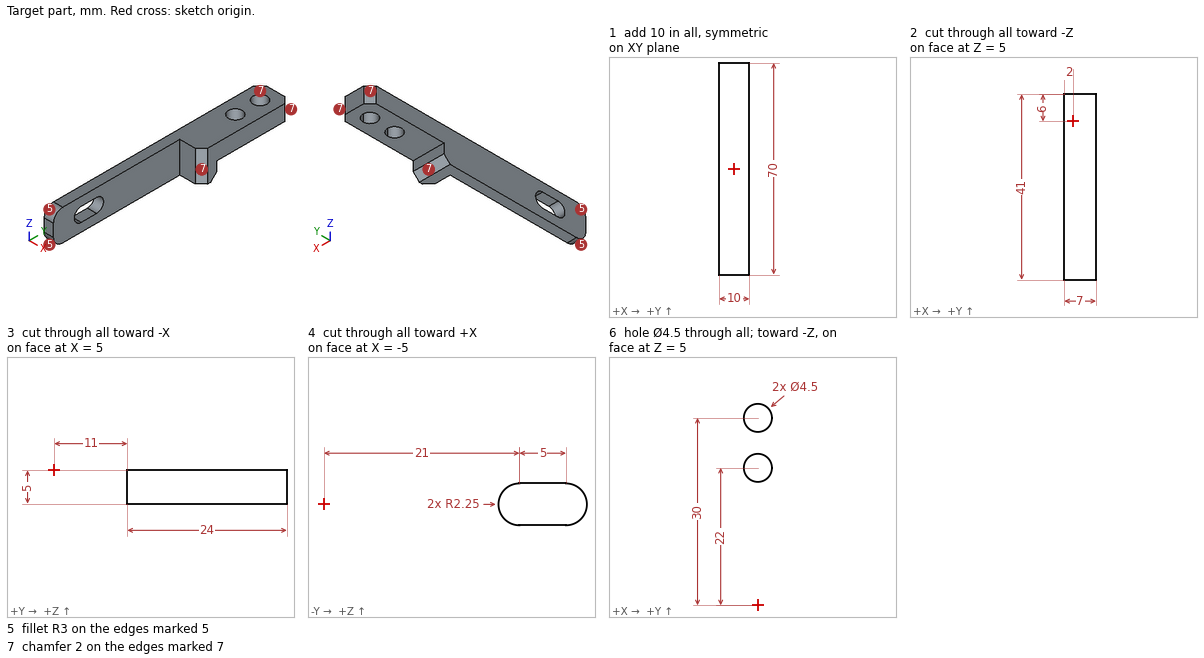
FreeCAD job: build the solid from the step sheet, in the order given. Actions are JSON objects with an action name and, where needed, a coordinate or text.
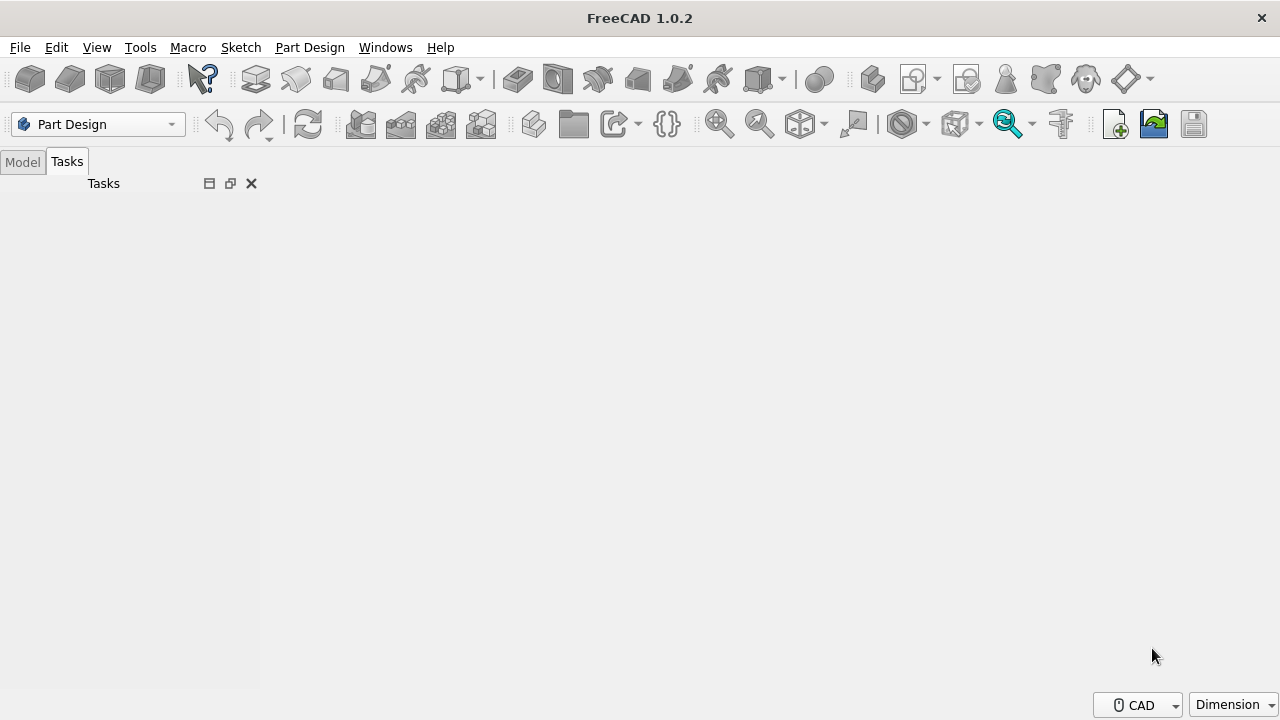
{"action": "key", "text": "ctrl+n"}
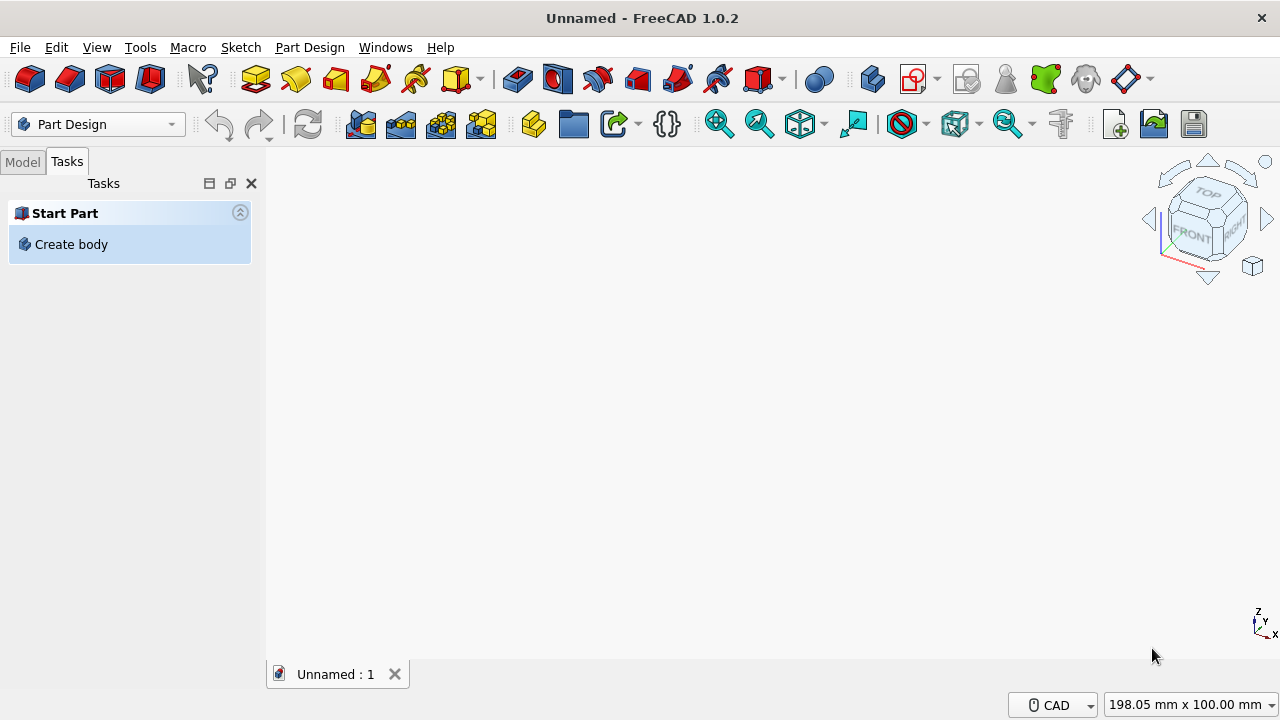
{"action": "left_click", "coordinate": [914, 80]}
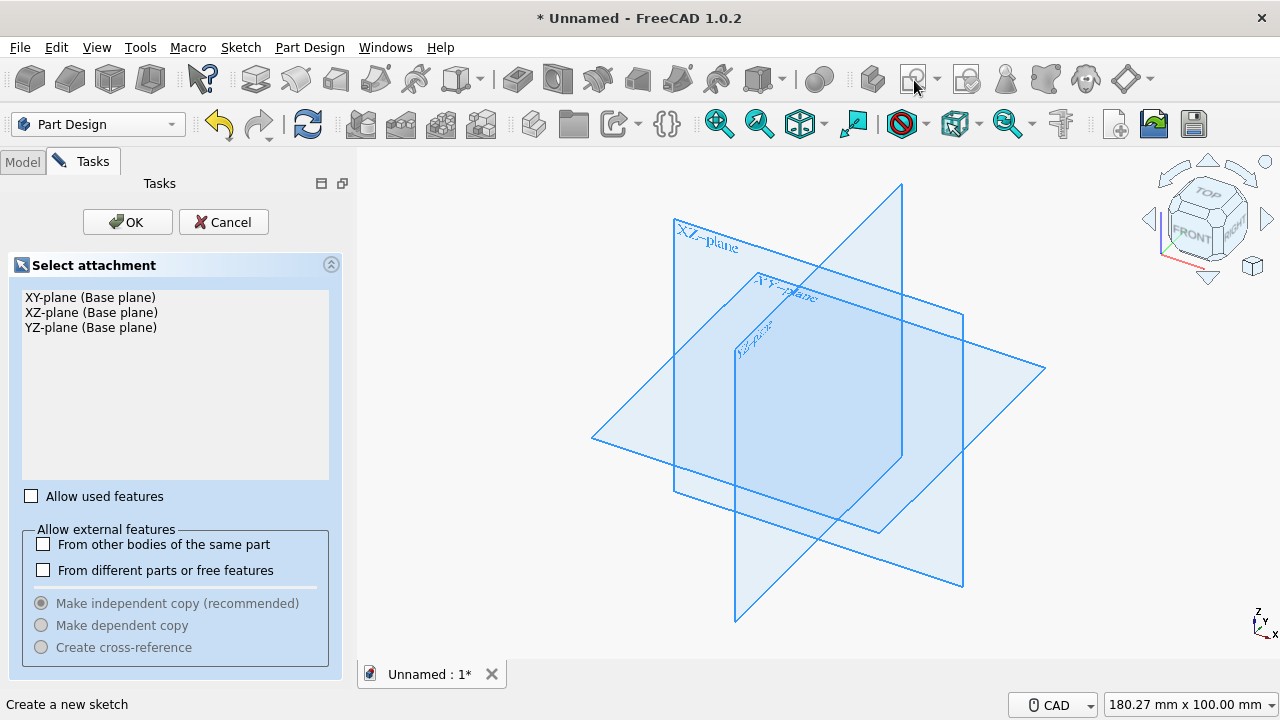
{"action": "left_click", "coordinate": [82, 298]}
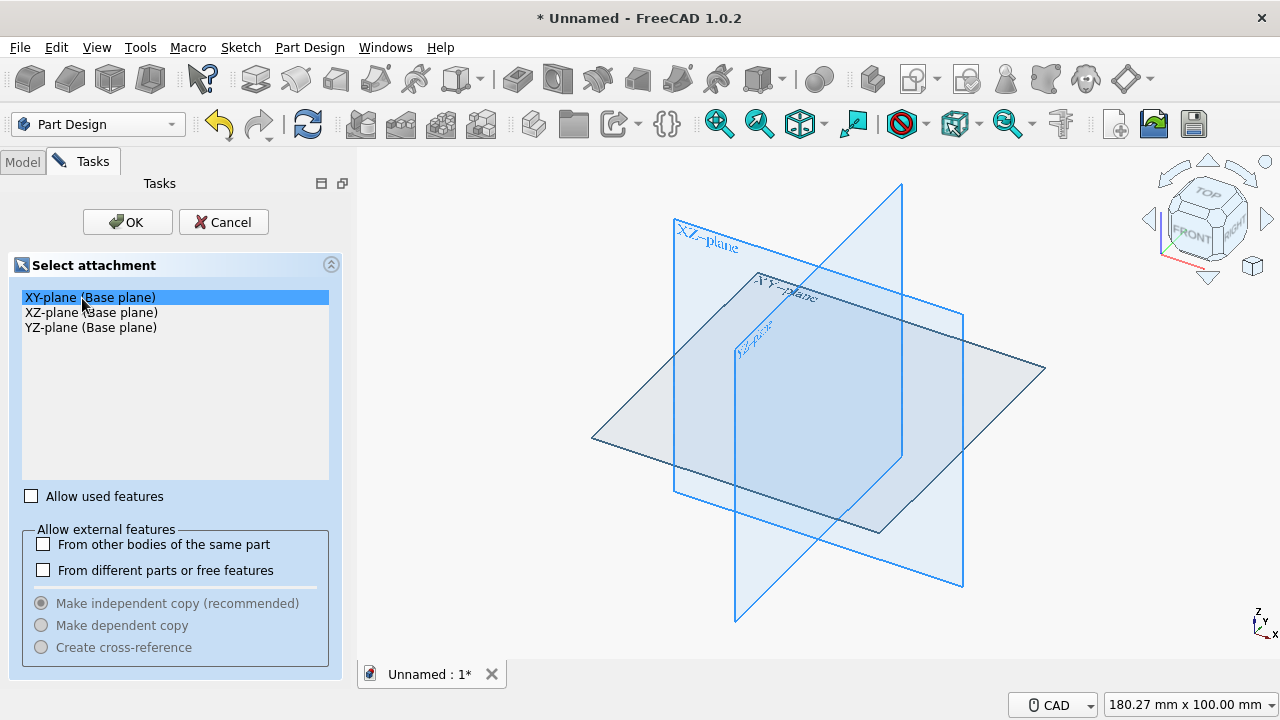
{"action": "left_click", "coordinate": [128, 222]}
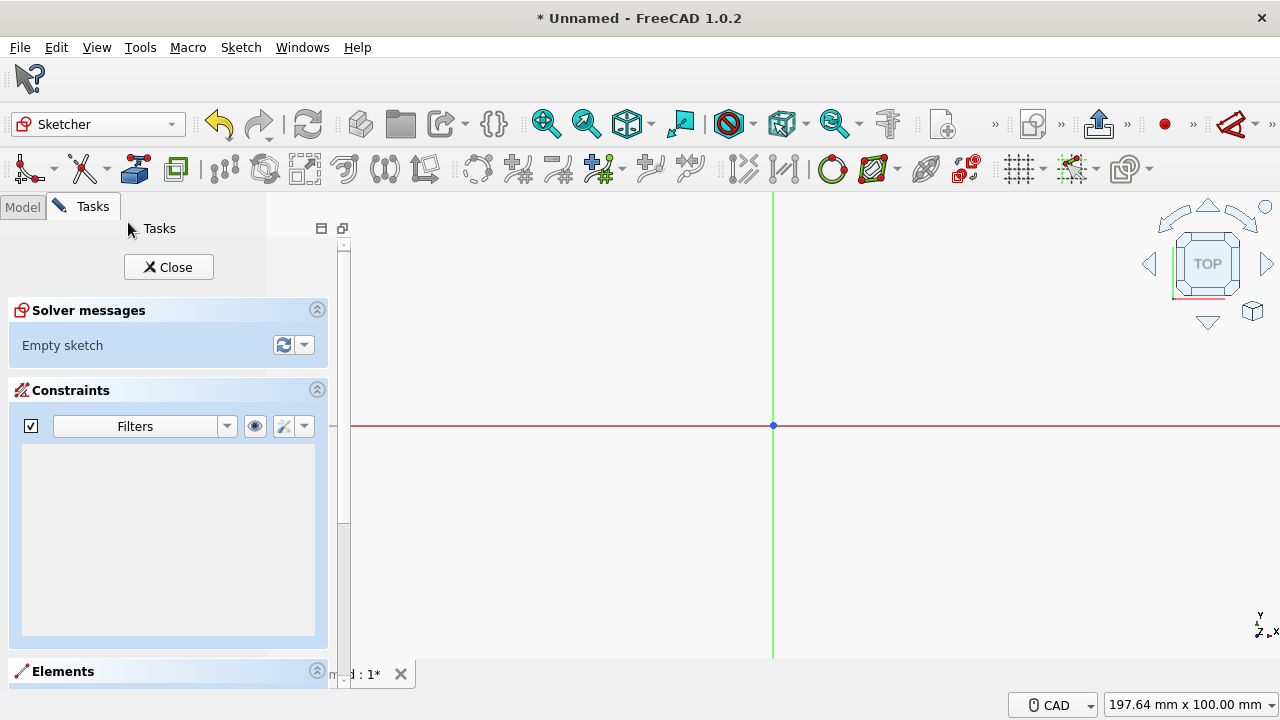
{"action": "key", "text": "g v"}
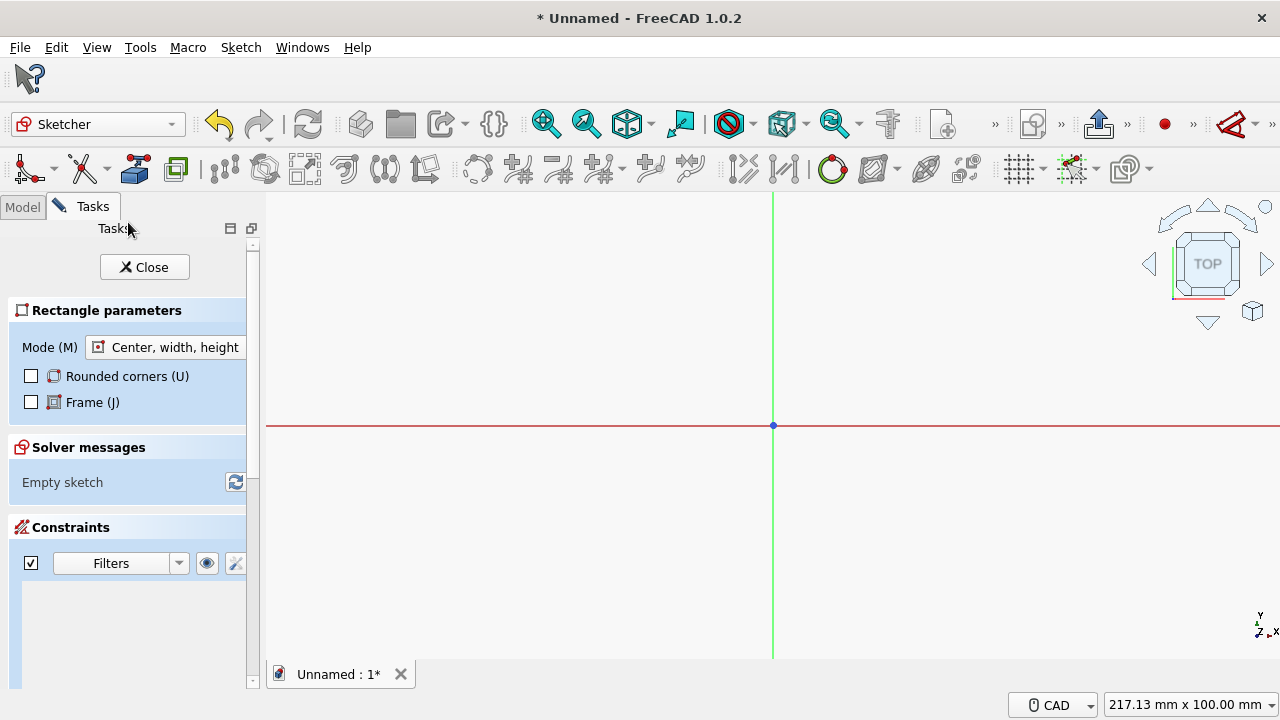
{"action": "left_click", "coordinate": [773, 426]}
{"action": "left_click", "coordinate": [796, 262]}
{"action": "key", "text": "Escape"}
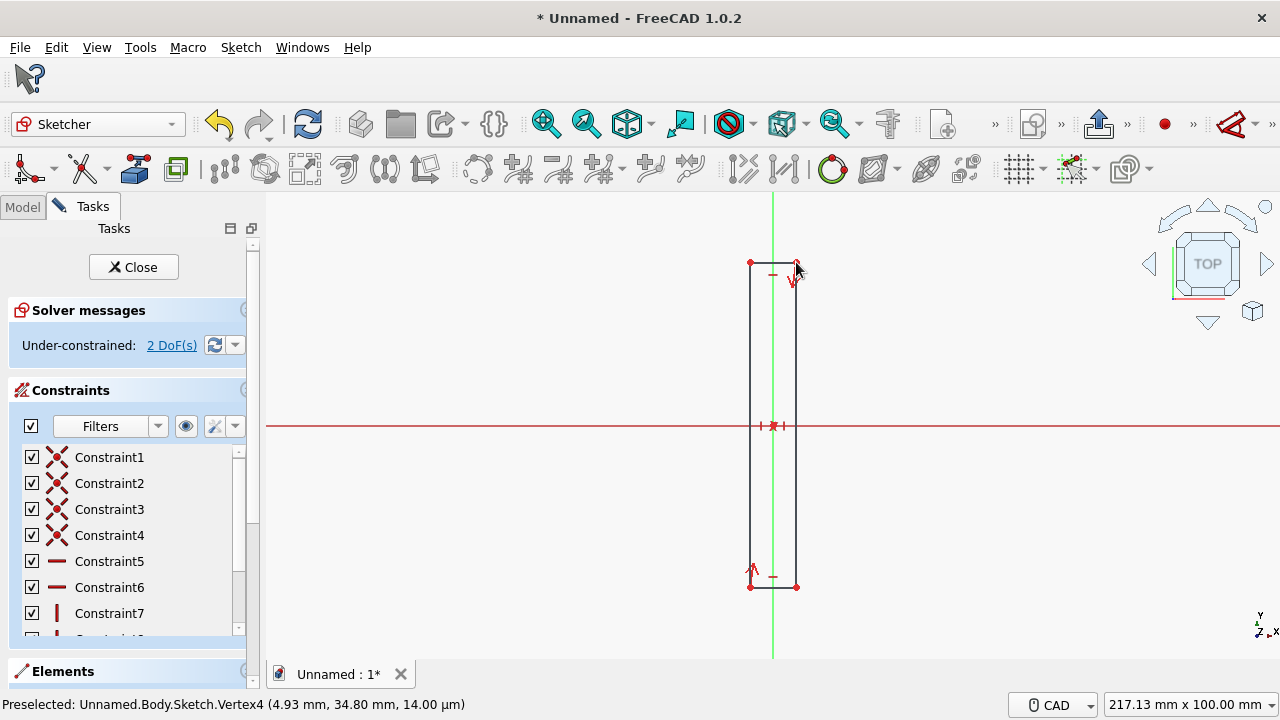
{"action": "key", "text": "d"}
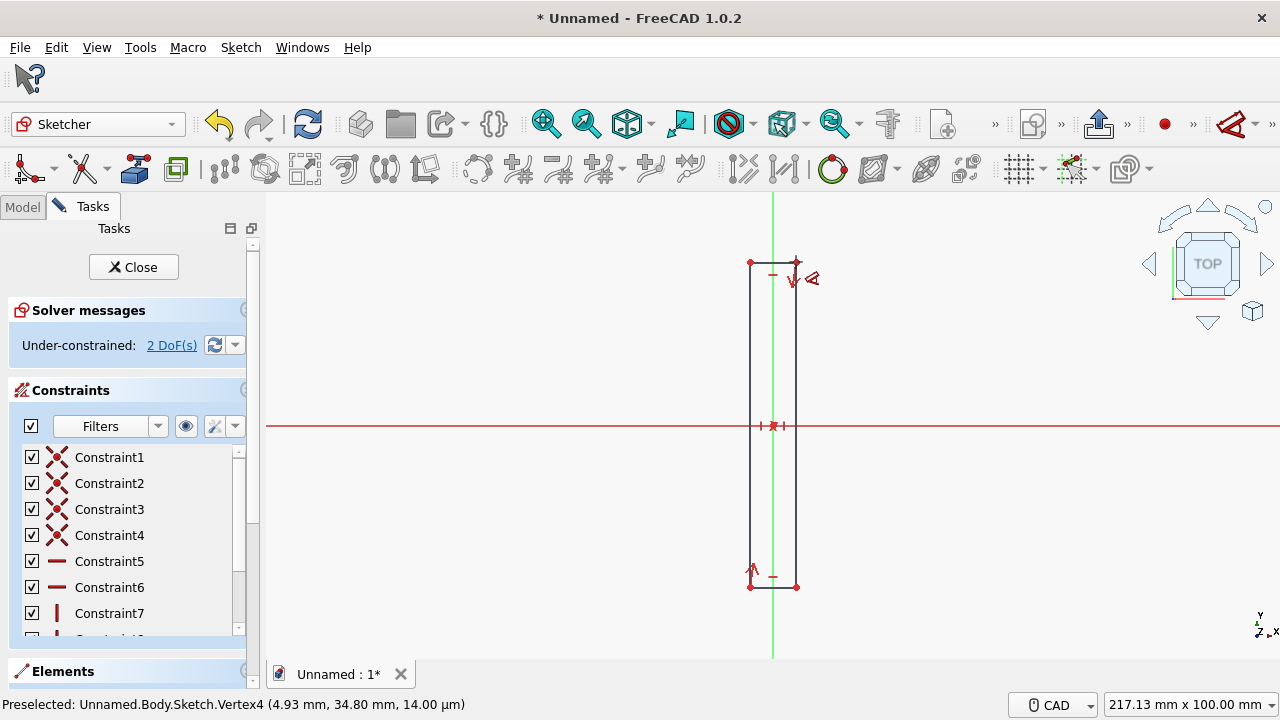
{"action": "scroll", "coordinate": [764, 588], "scroll_direction": "up", "scroll_amount": 3}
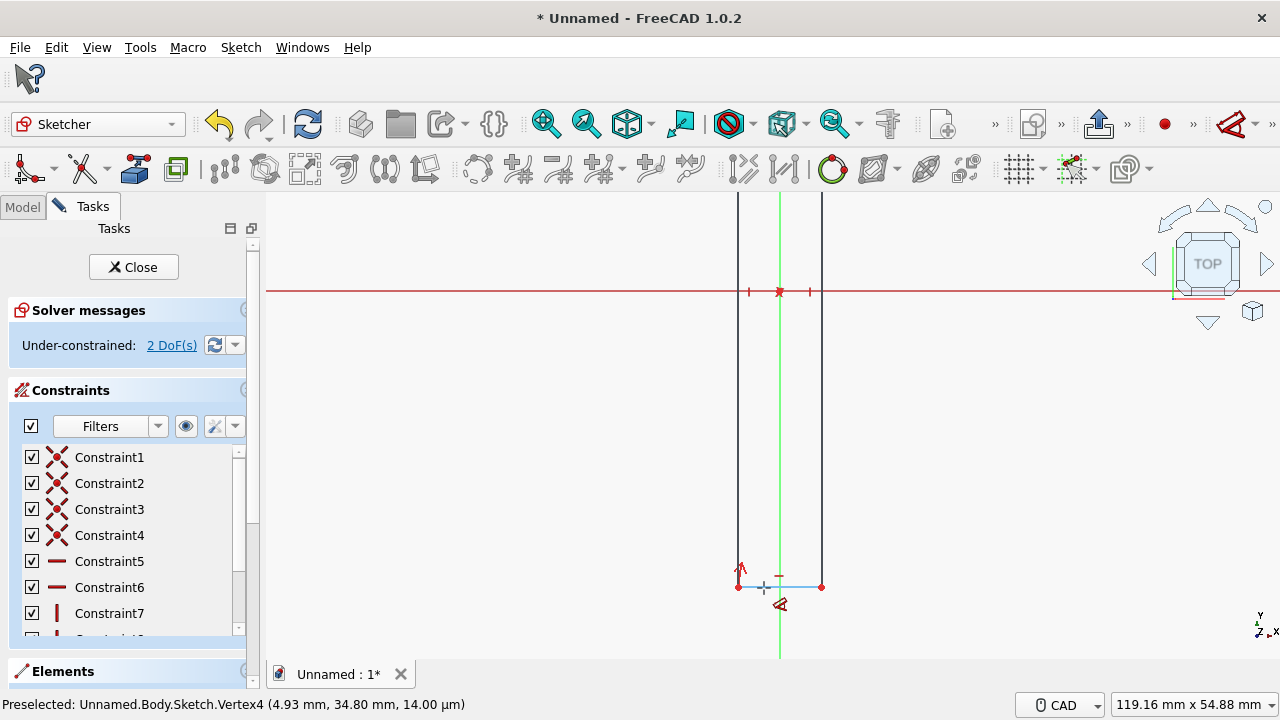
{"action": "left_click", "coordinate": [763, 587]}
{"action": "left_click", "coordinate": [761, 621]}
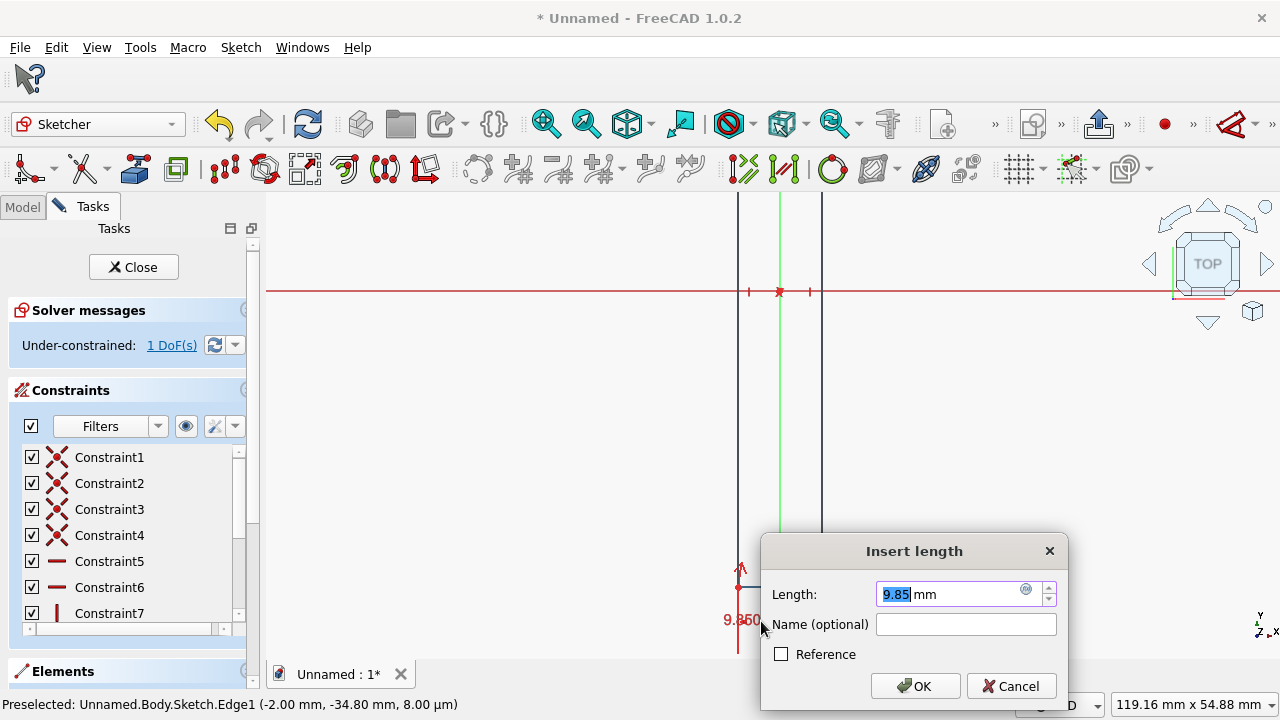
{"action": "type", "text": "10"}
{"action": "key", "text": "Return"}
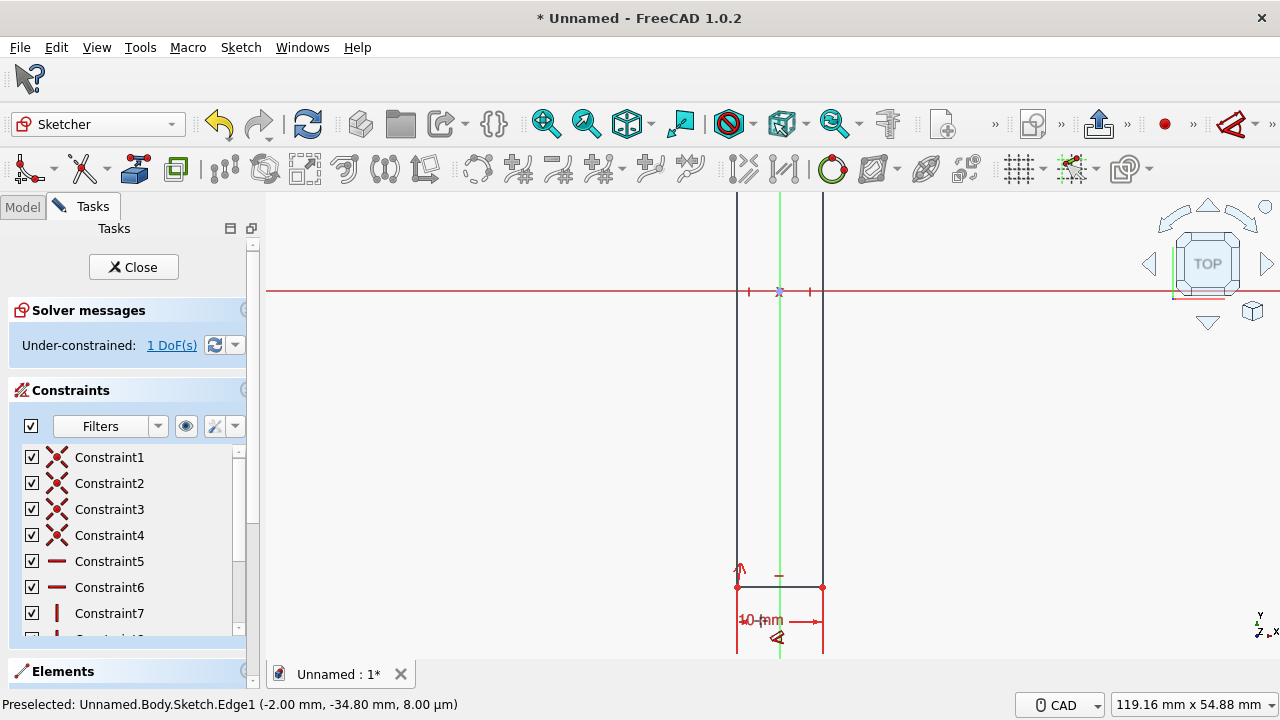
{"action": "left_click", "coordinate": [823, 410]}
{"action": "left_click", "coordinate": [857, 404]}